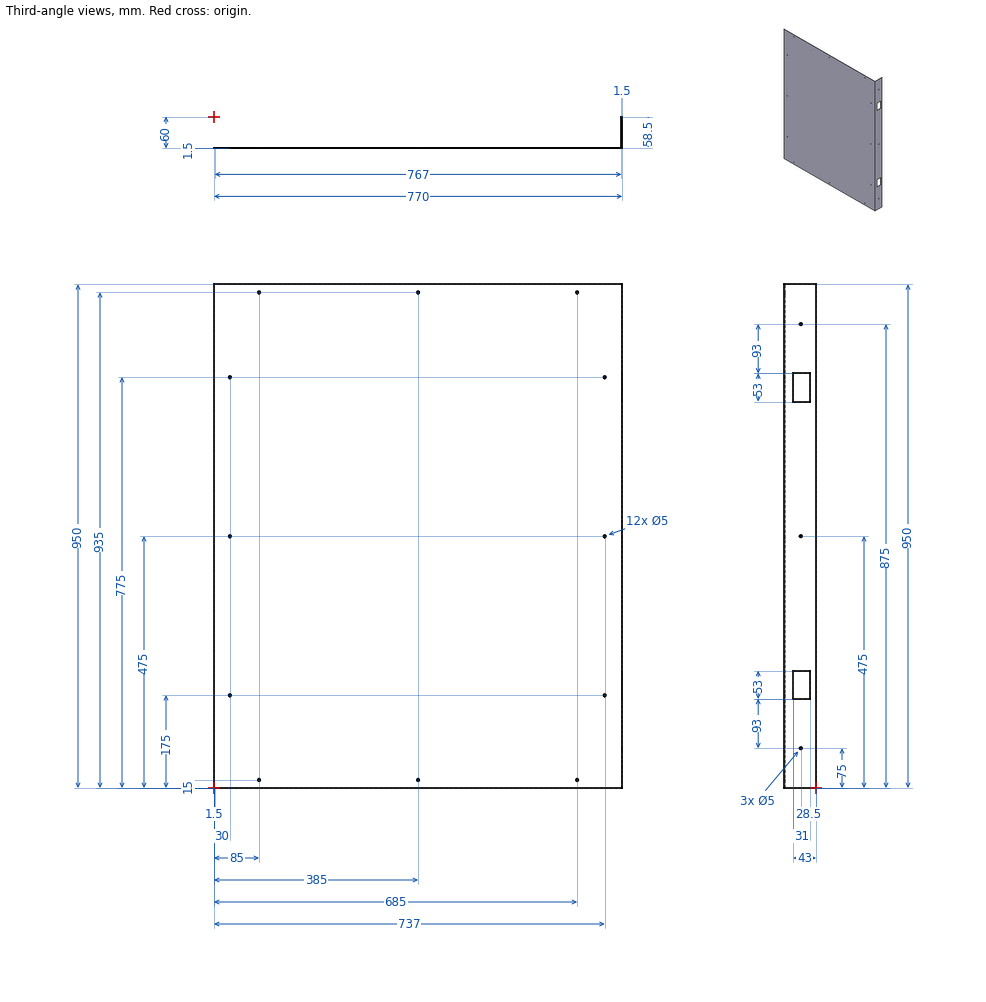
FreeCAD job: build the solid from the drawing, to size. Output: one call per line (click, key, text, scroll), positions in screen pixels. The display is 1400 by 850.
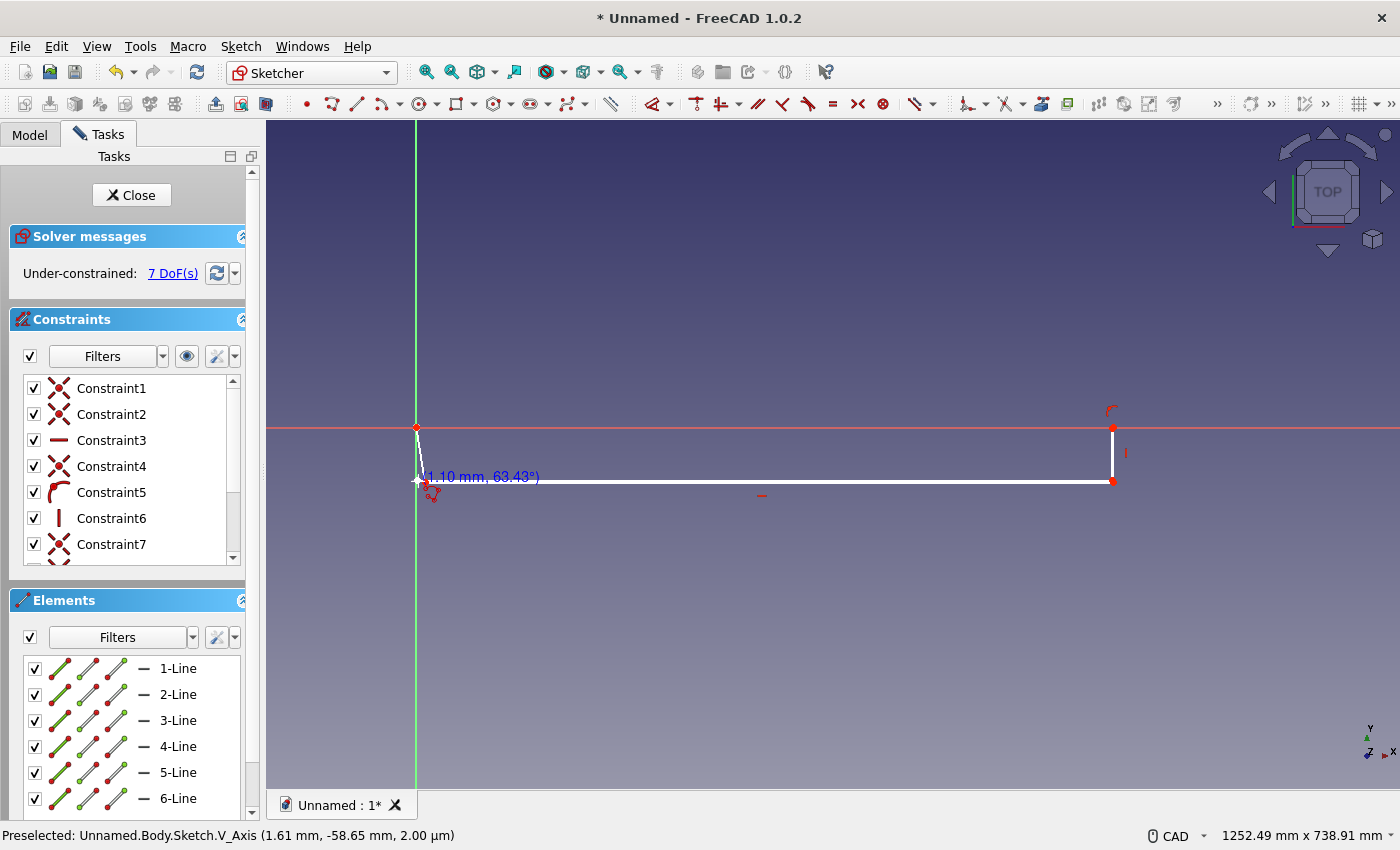
scroll(418, 428, up, 13)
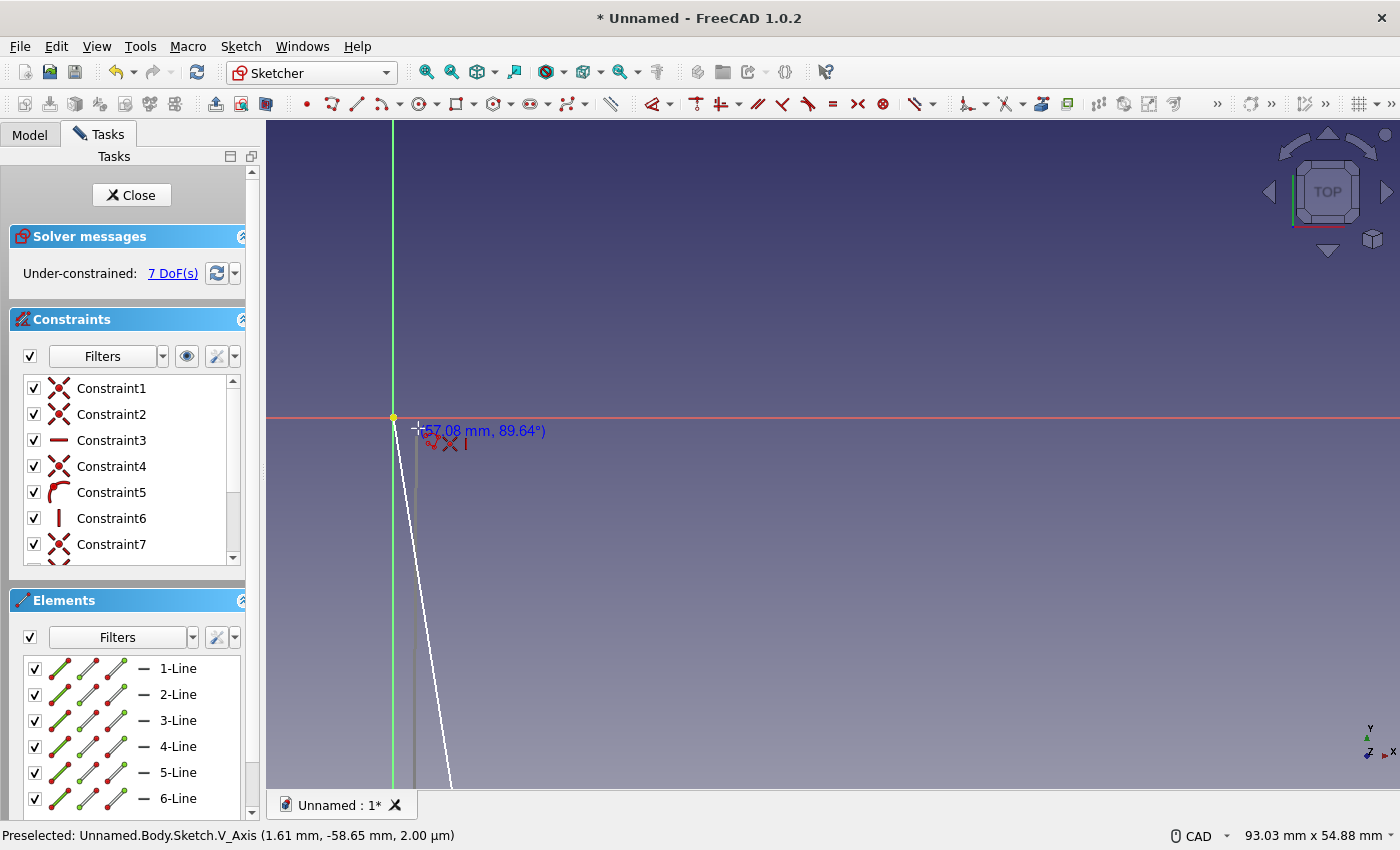
click(412, 427)
click(393, 418)
key(Escape)
key(Escape)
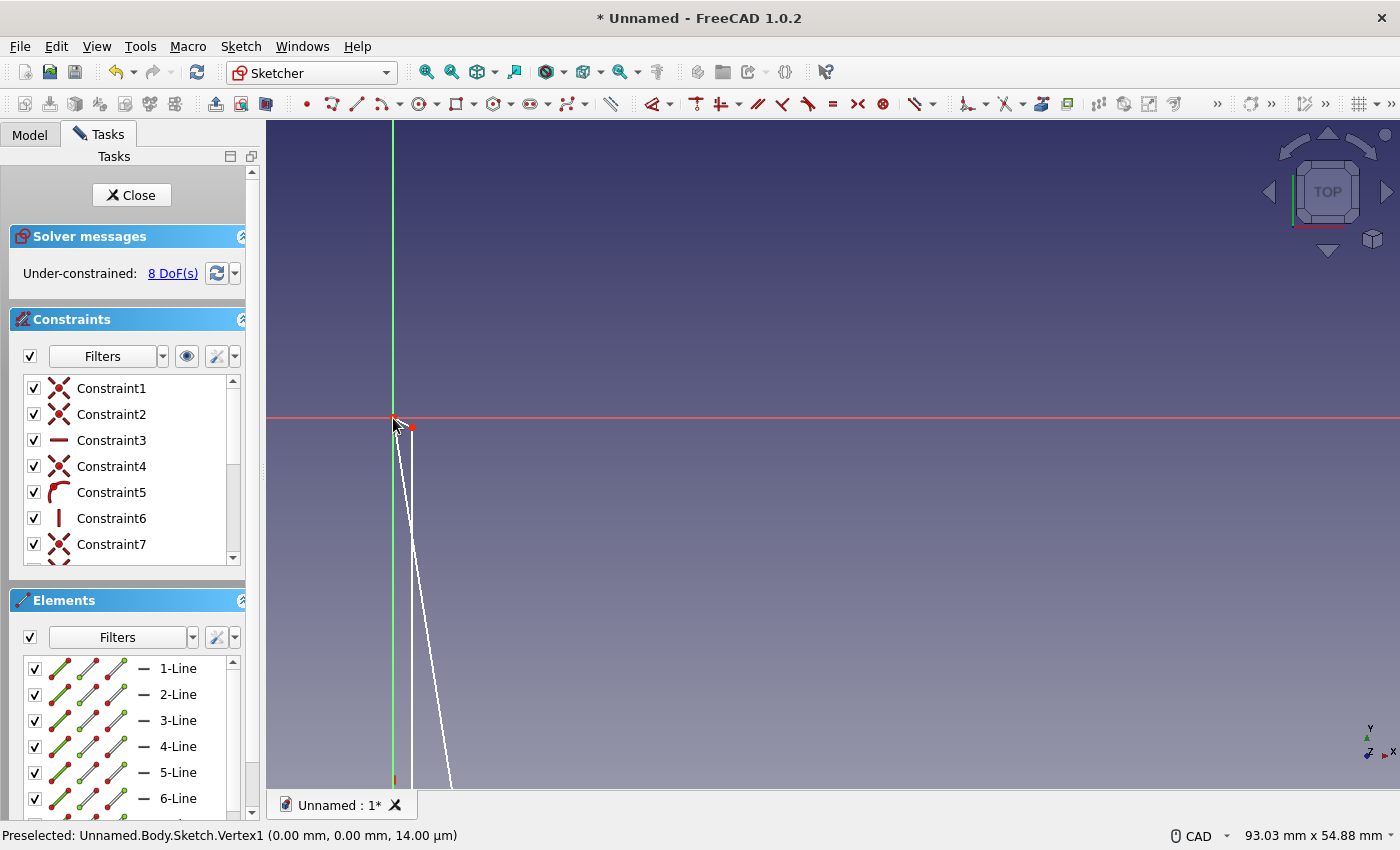
click(429, 641)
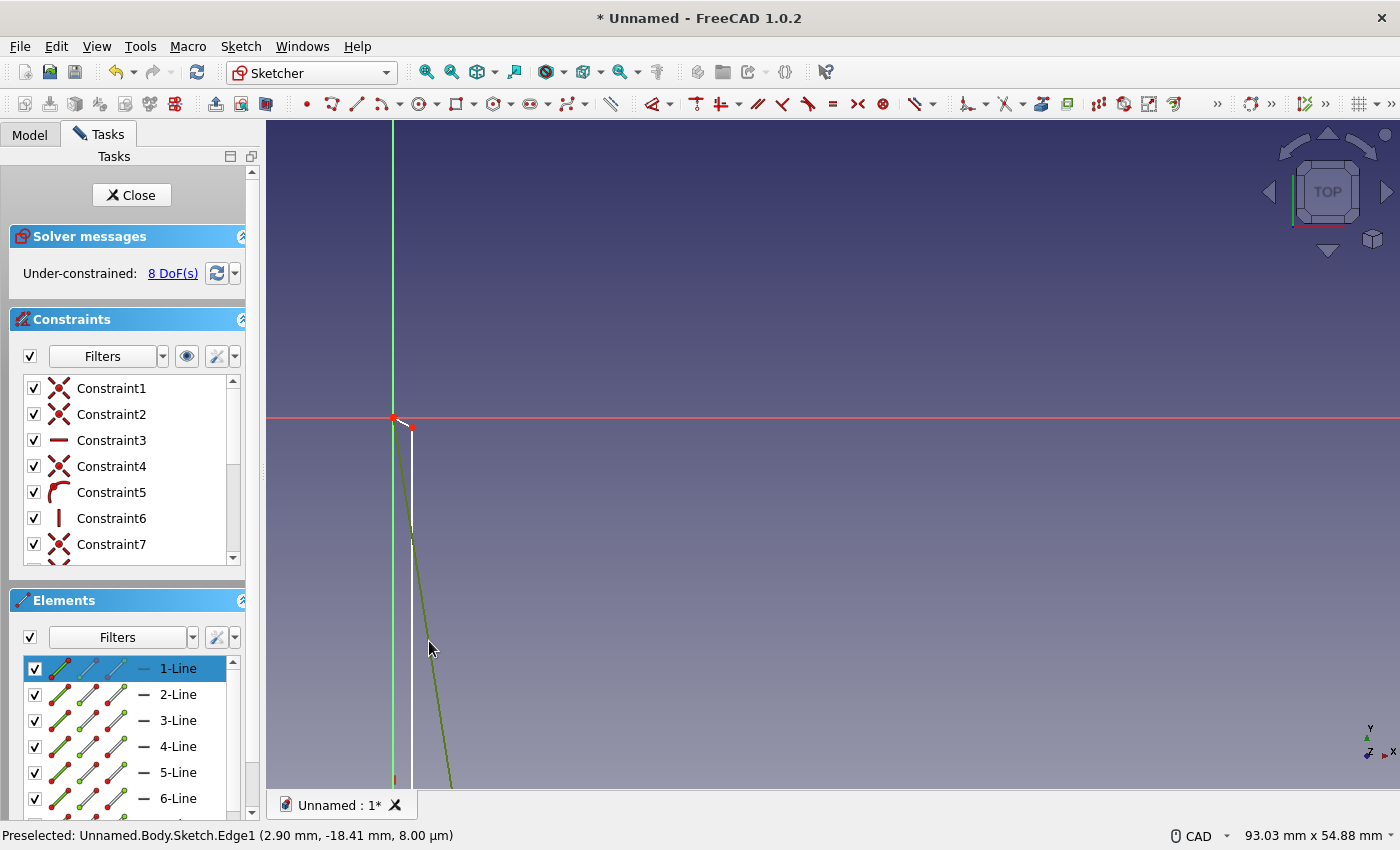
key(v)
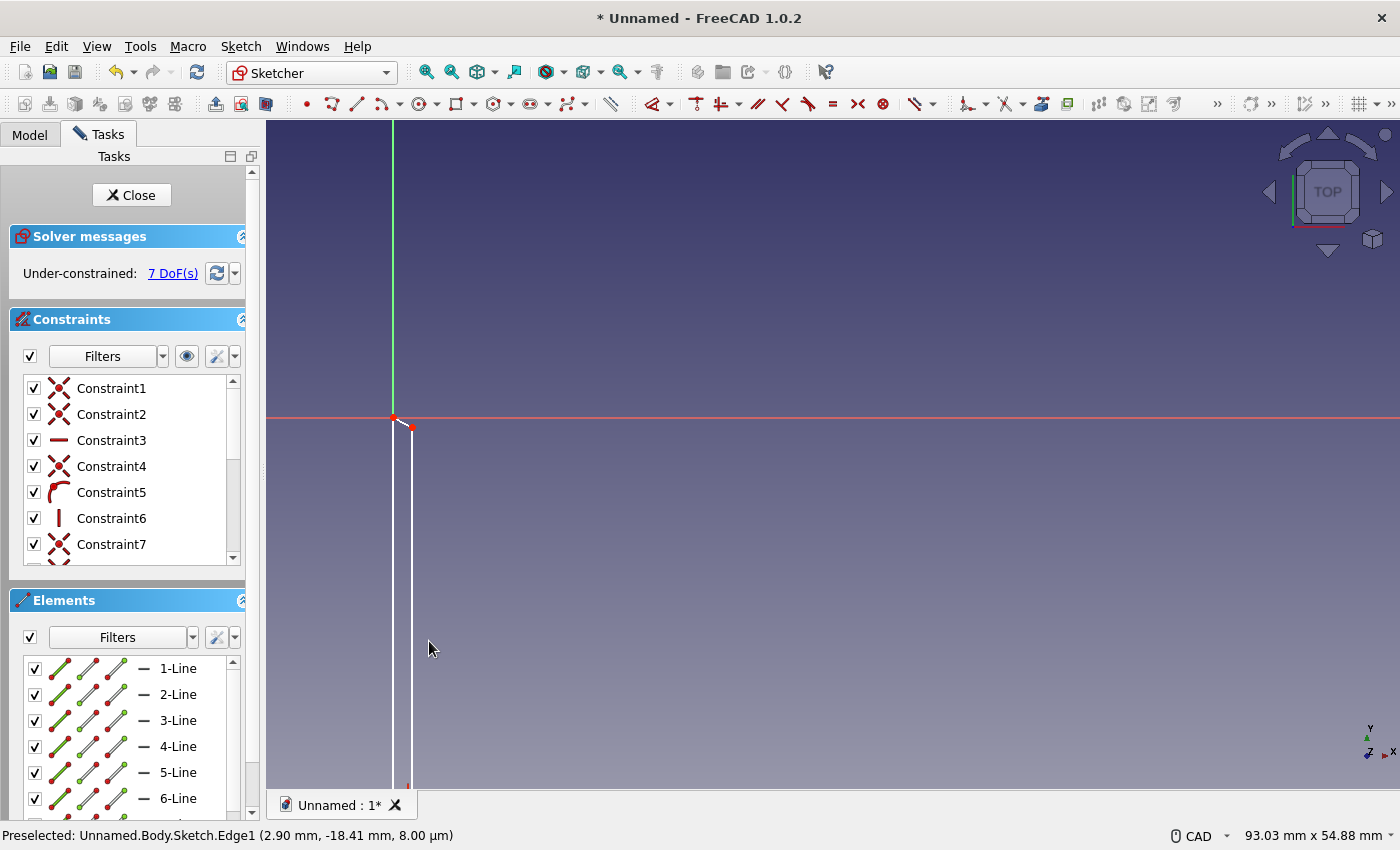
scroll(418, 428, down, 13)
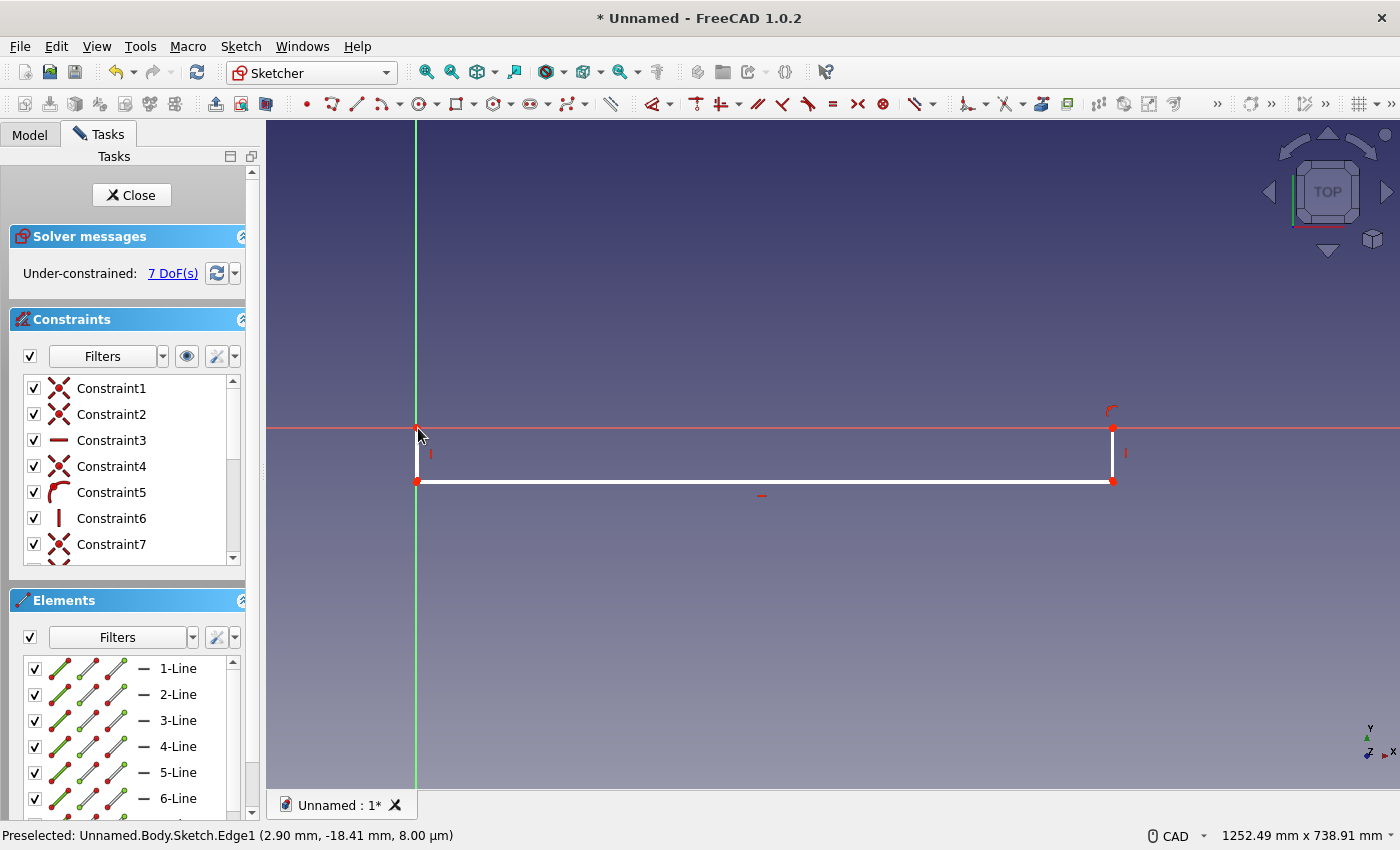
scroll(1112, 428, up, 14)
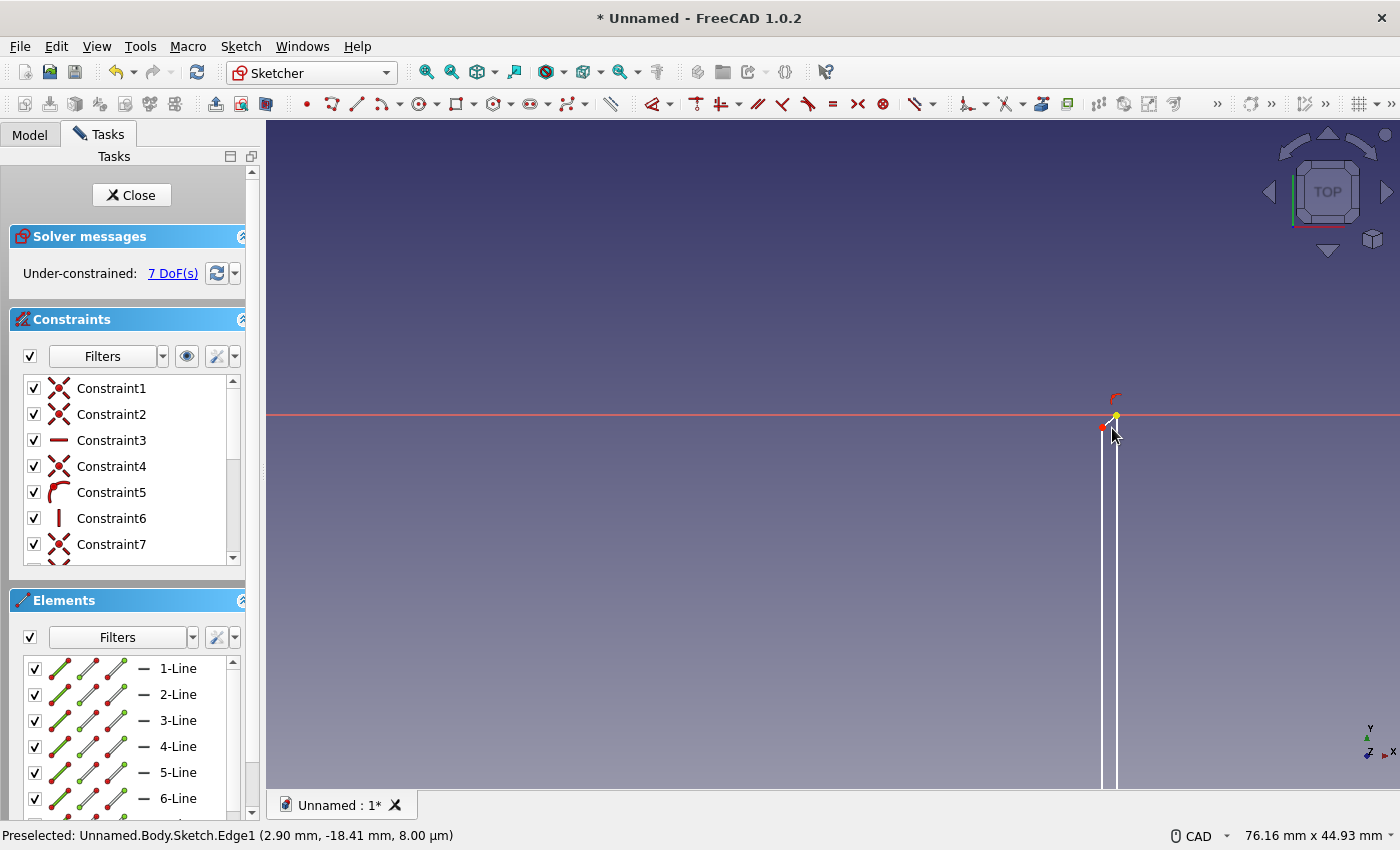
click(1108, 423)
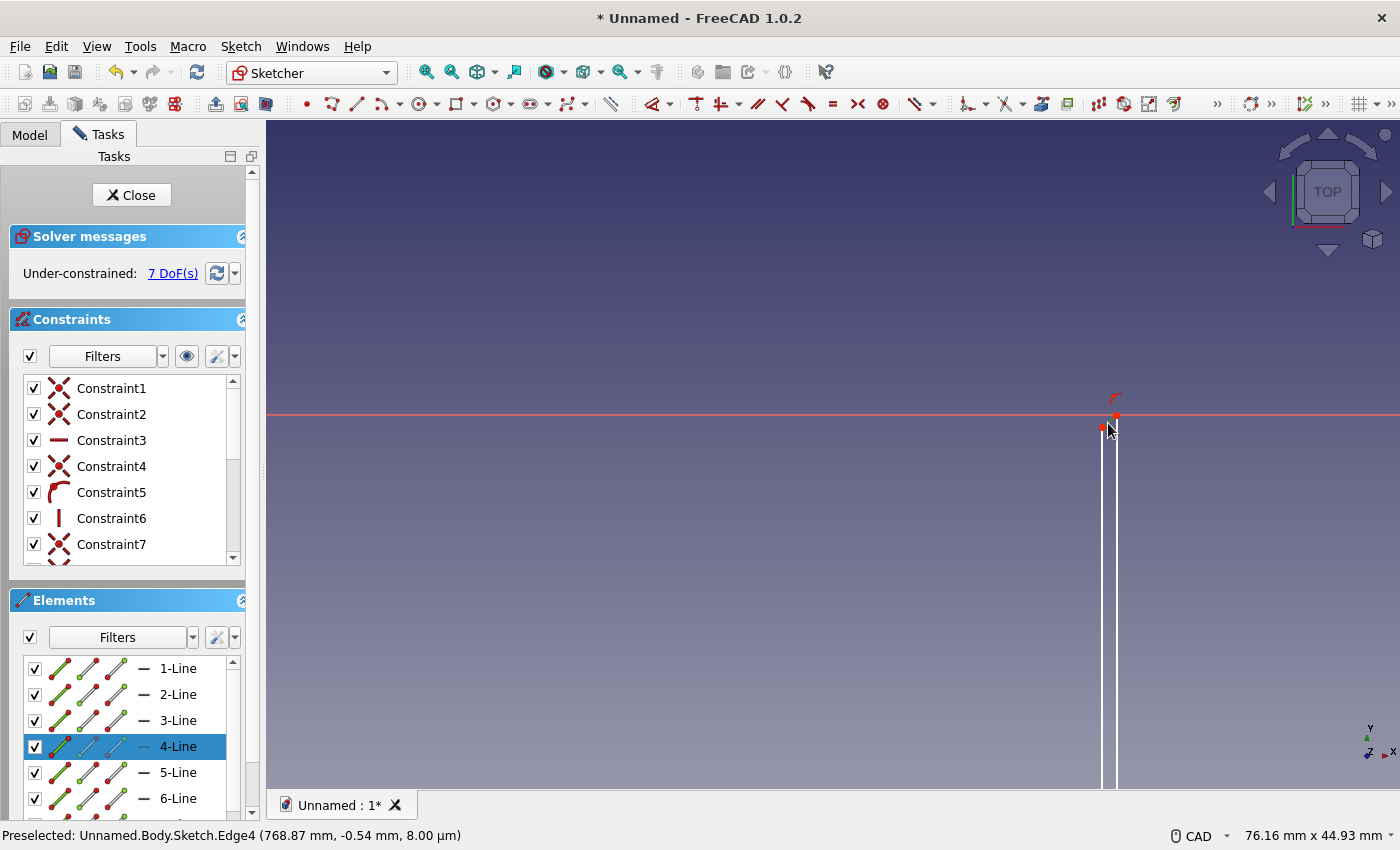
key(h)